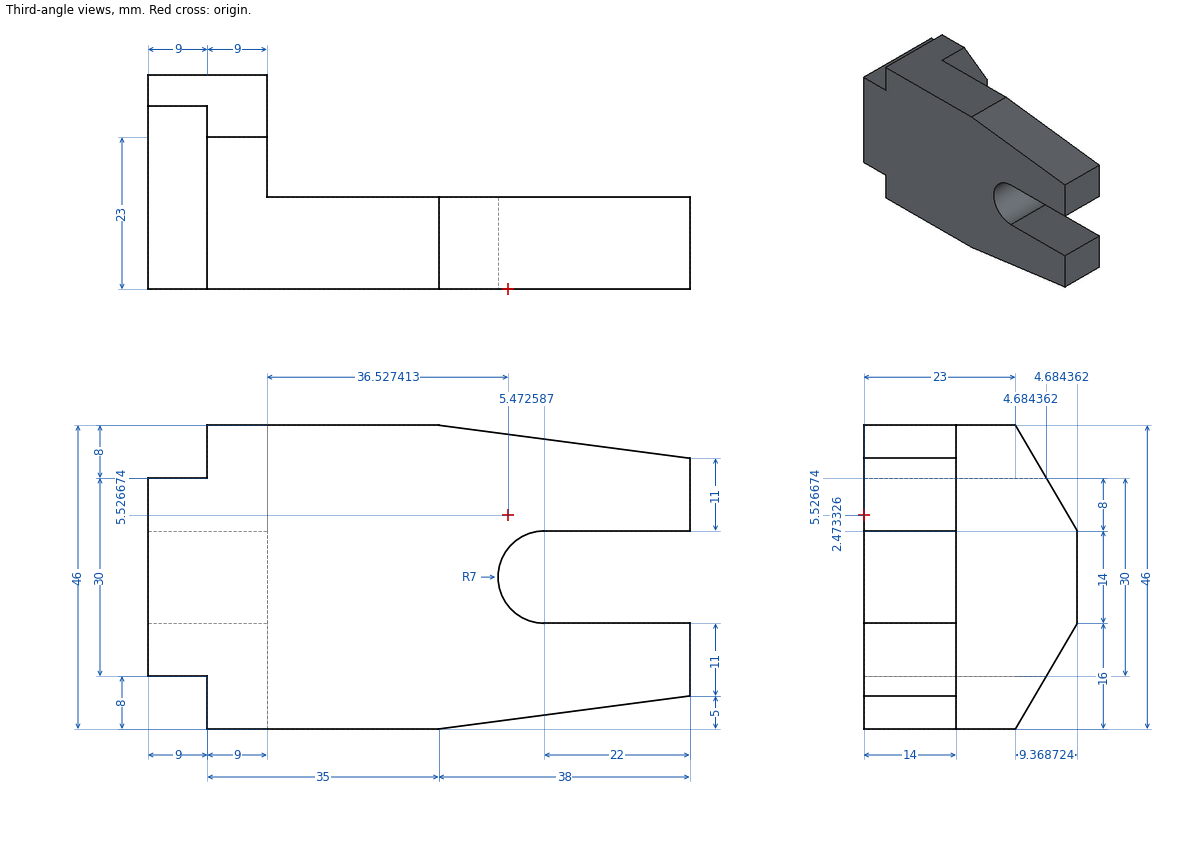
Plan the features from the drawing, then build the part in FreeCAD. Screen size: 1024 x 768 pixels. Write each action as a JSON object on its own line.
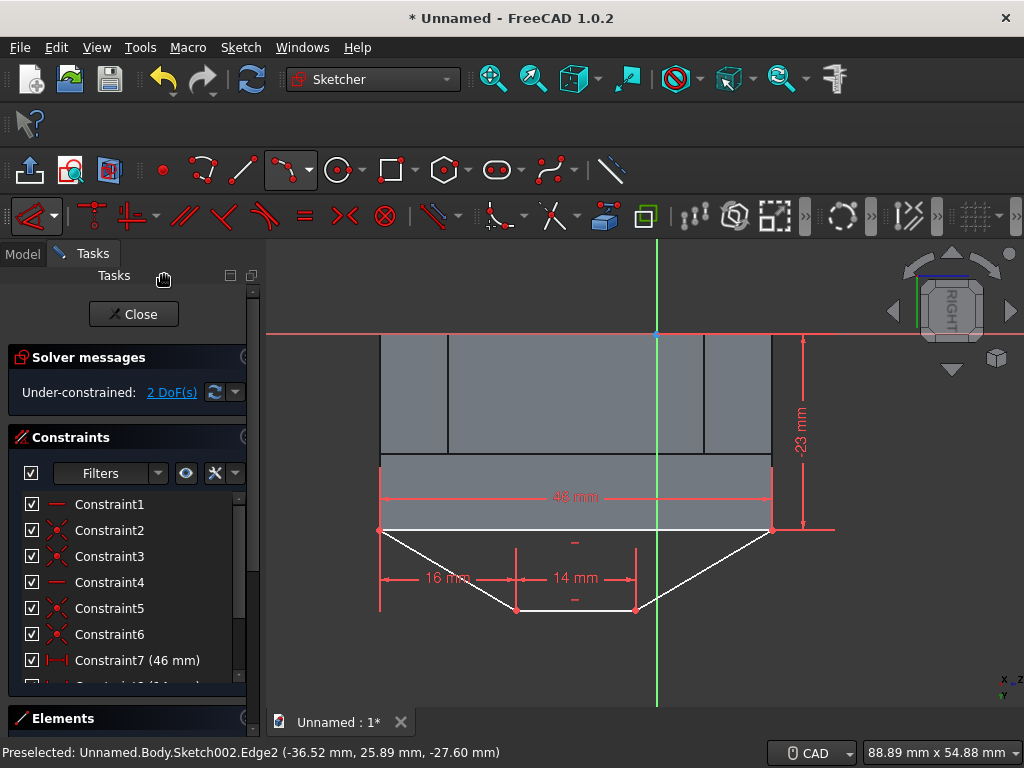
{"action": "scroll", "coordinate": [636, 611], "scroll_direction": "up", "scroll_amount": 4}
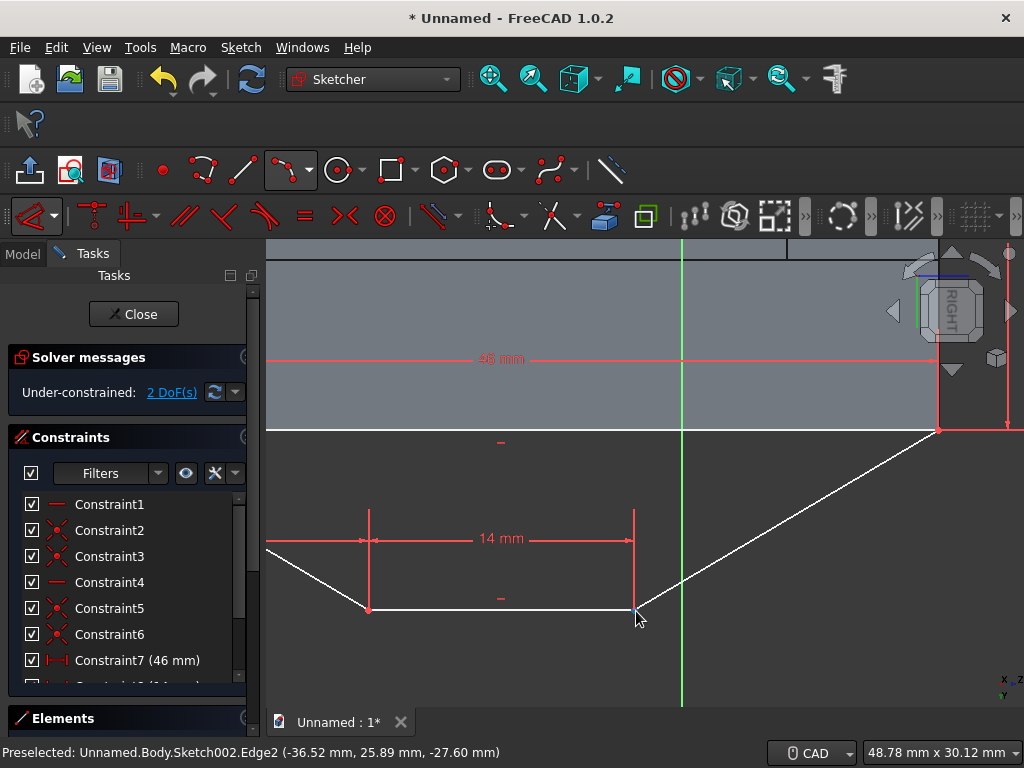
{"action": "left_click", "coordinate": [634, 610]}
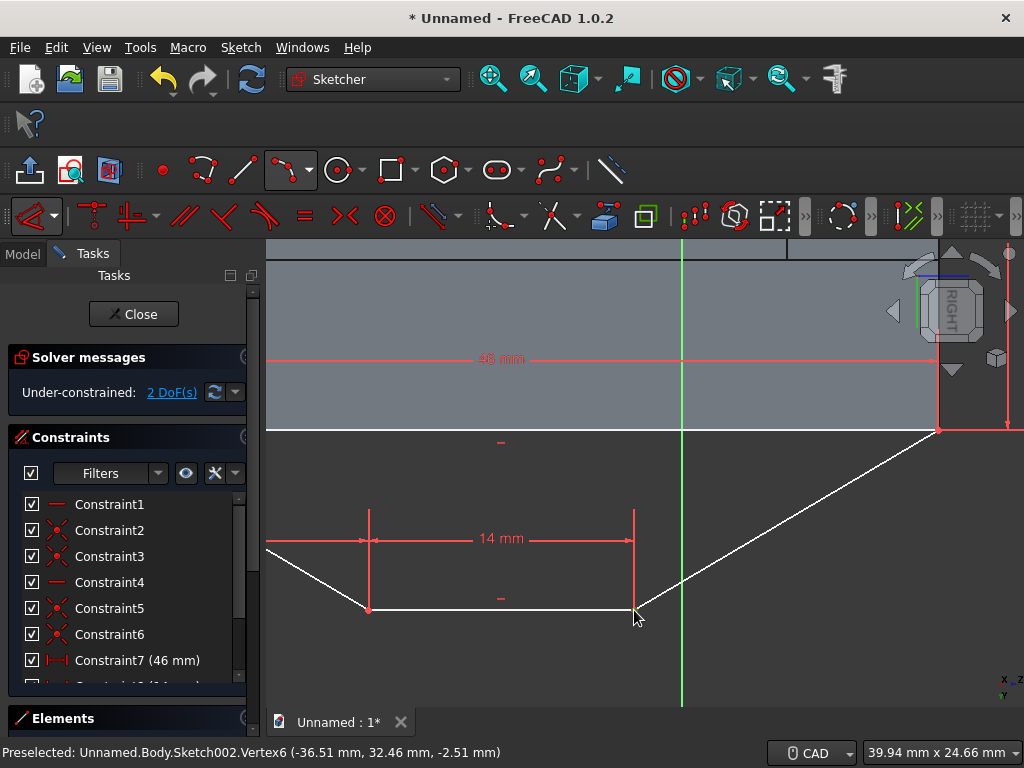
{"action": "left_click", "coordinate": [56, 216]}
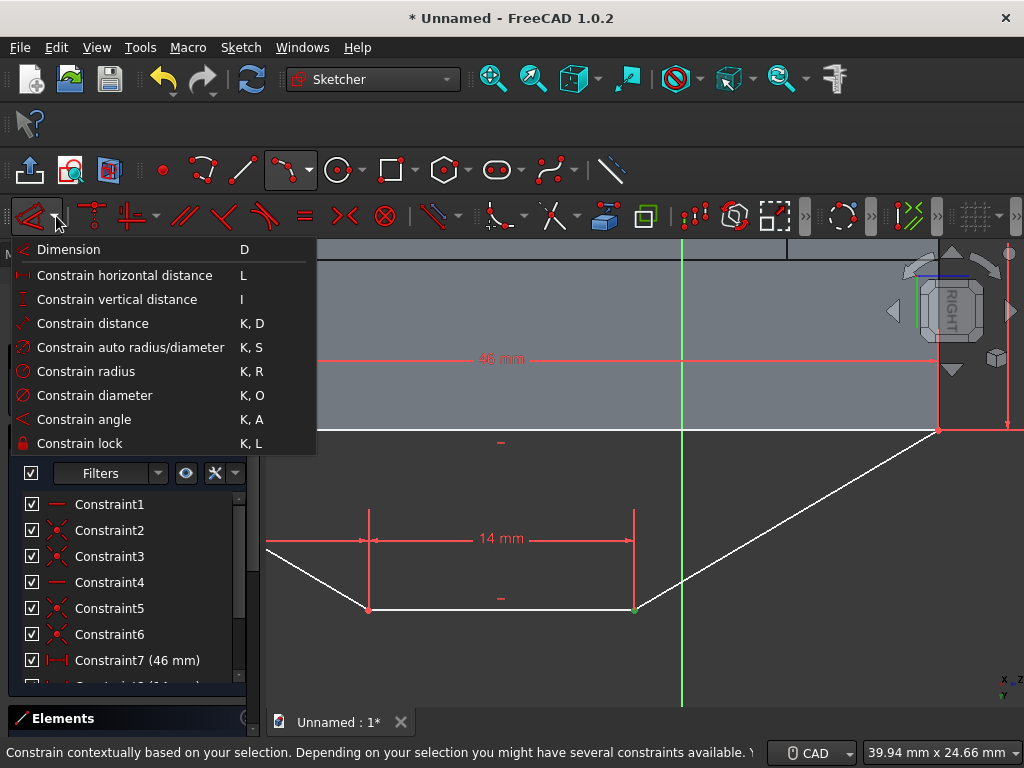
{"action": "left_click", "coordinate": [164, 275]}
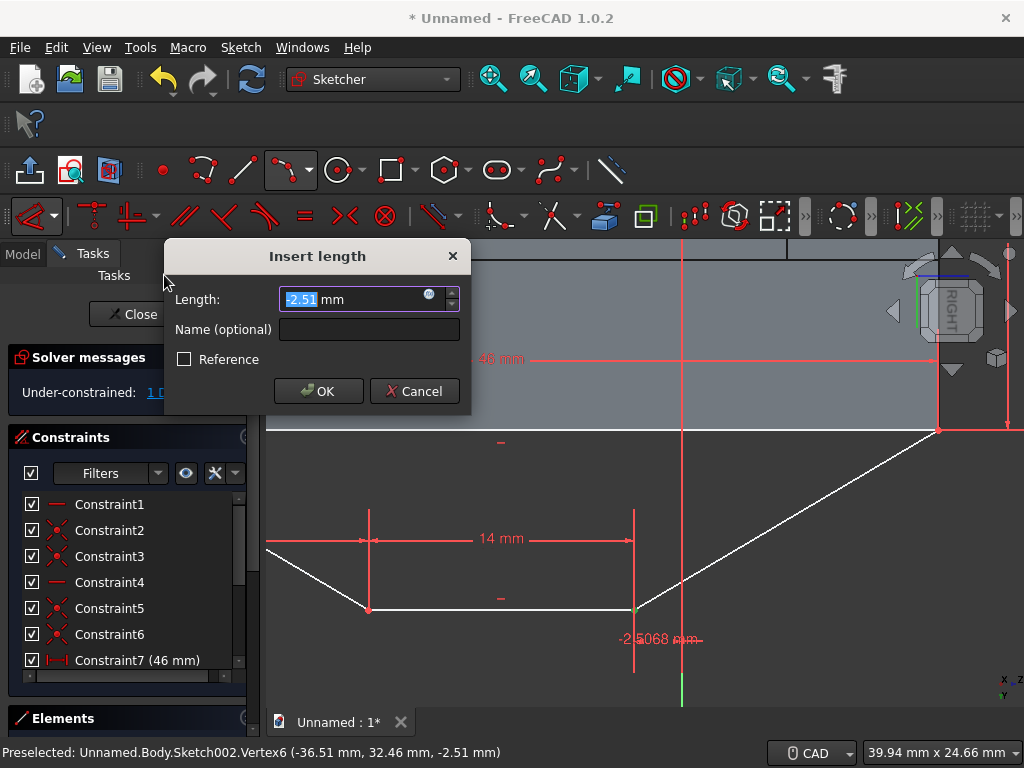
{"action": "type", "text": "-2.473326"}
{"action": "key", "text": "Return"}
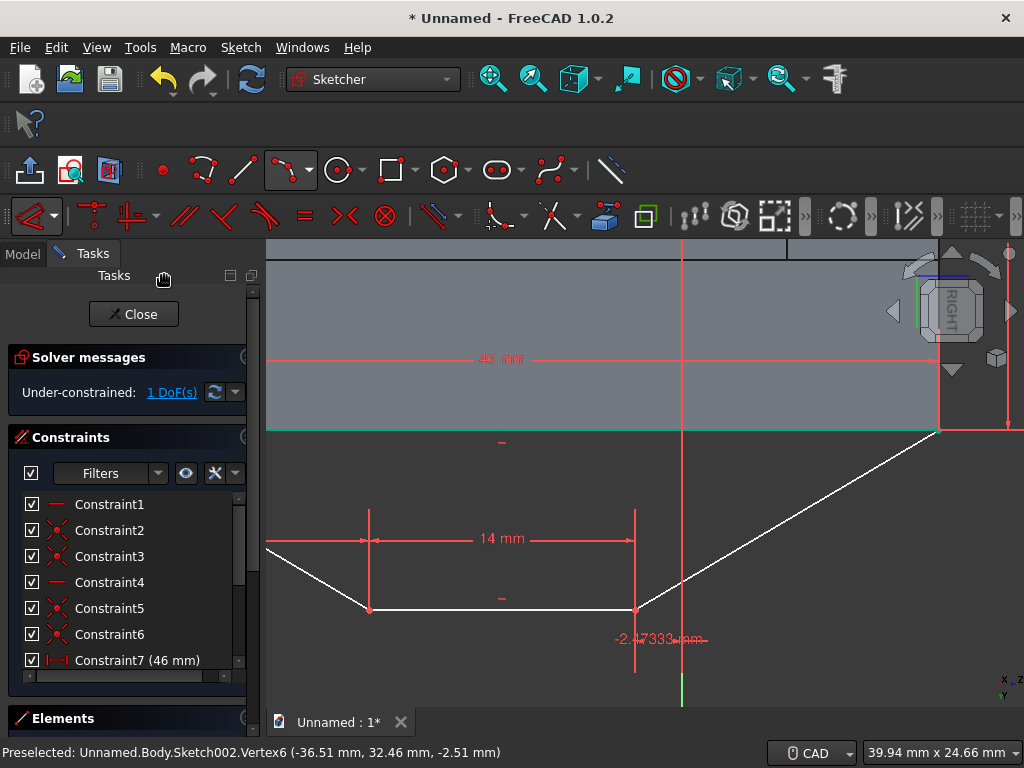
{"action": "left_click", "coordinate": [309, 574]}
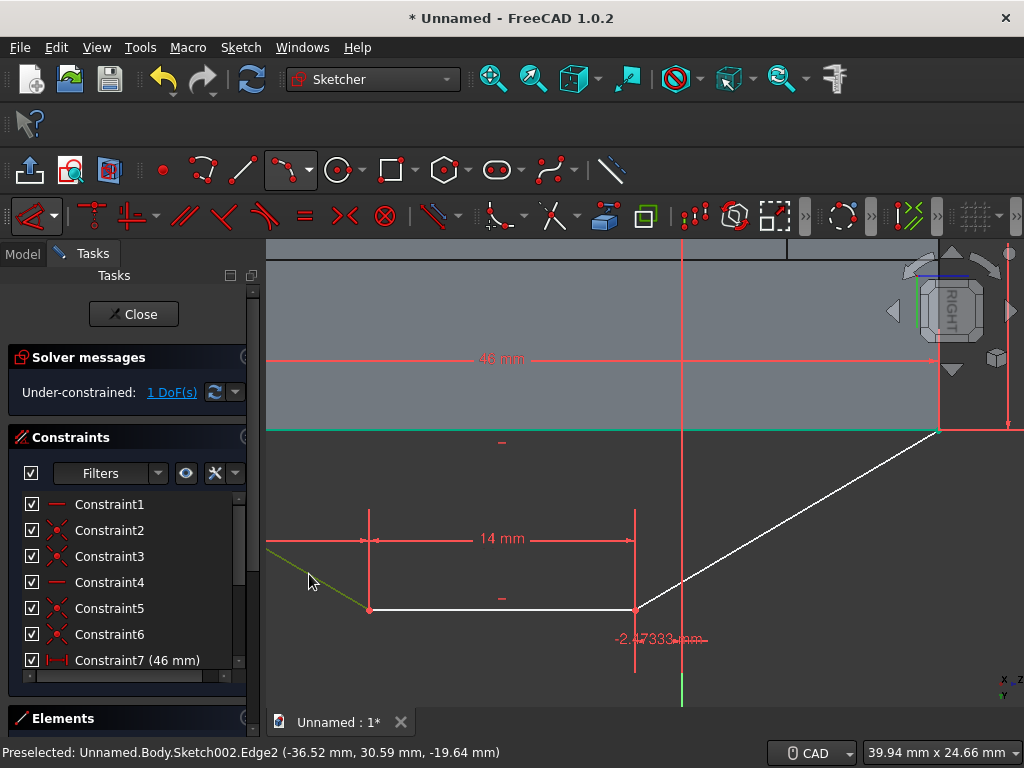
{"action": "key", "text": "i"}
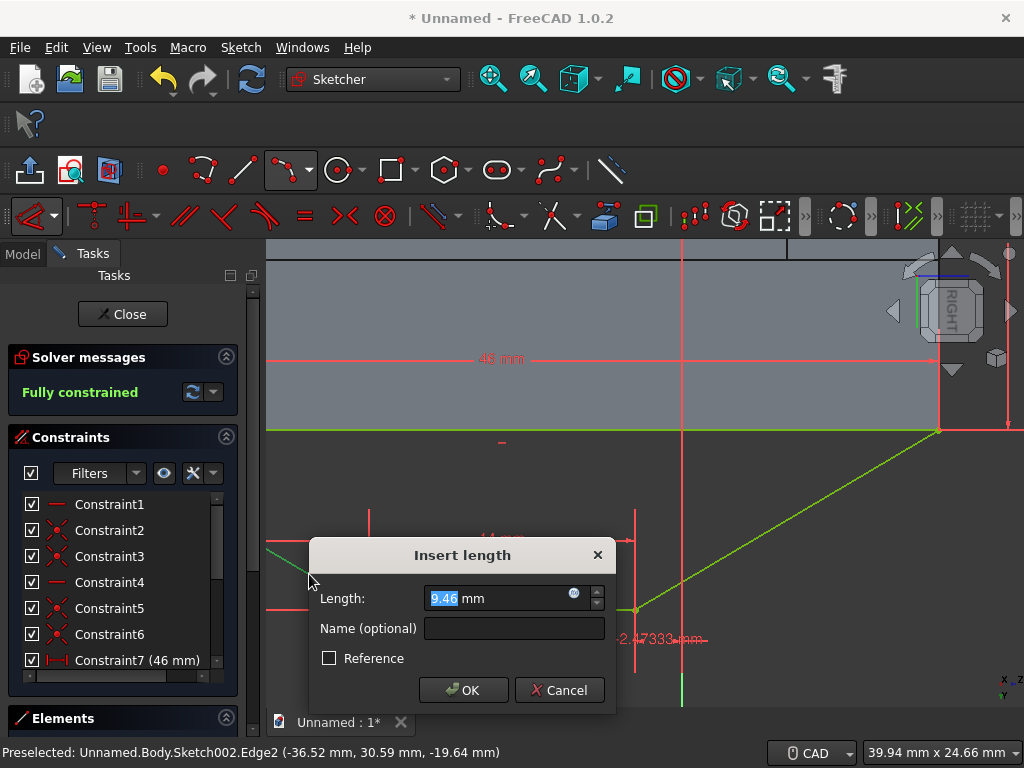
{"action": "type", "text": "9.368724"}
{"action": "key", "text": "Return"}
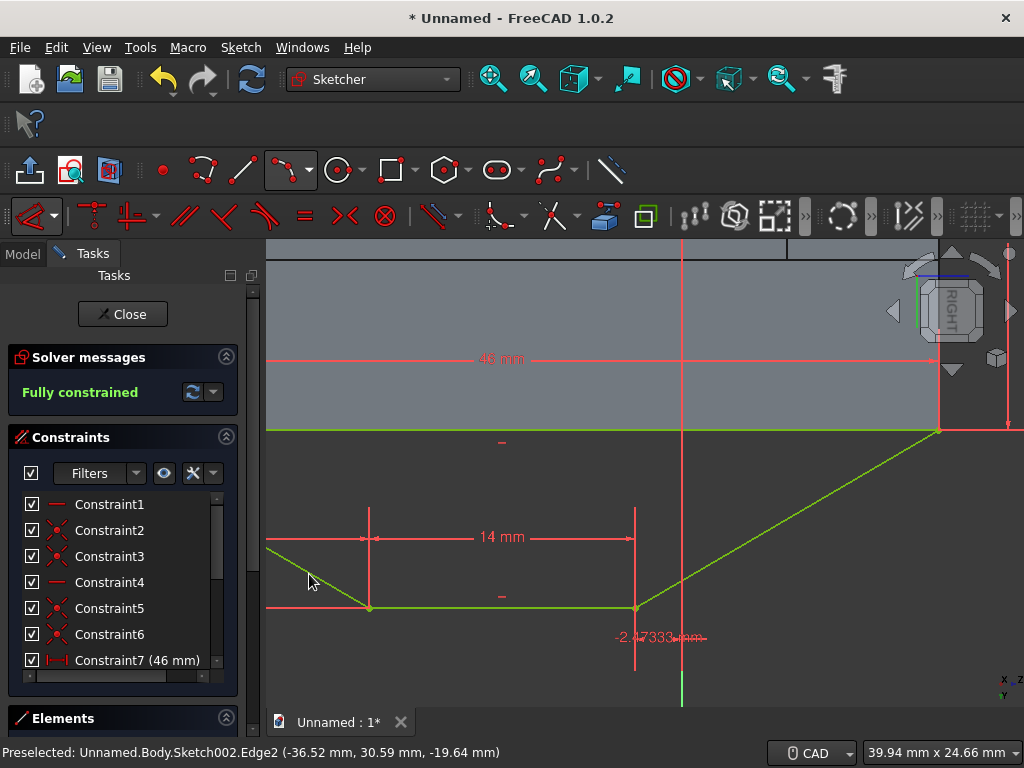
{"action": "left_click", "coordinate": [123, 314]}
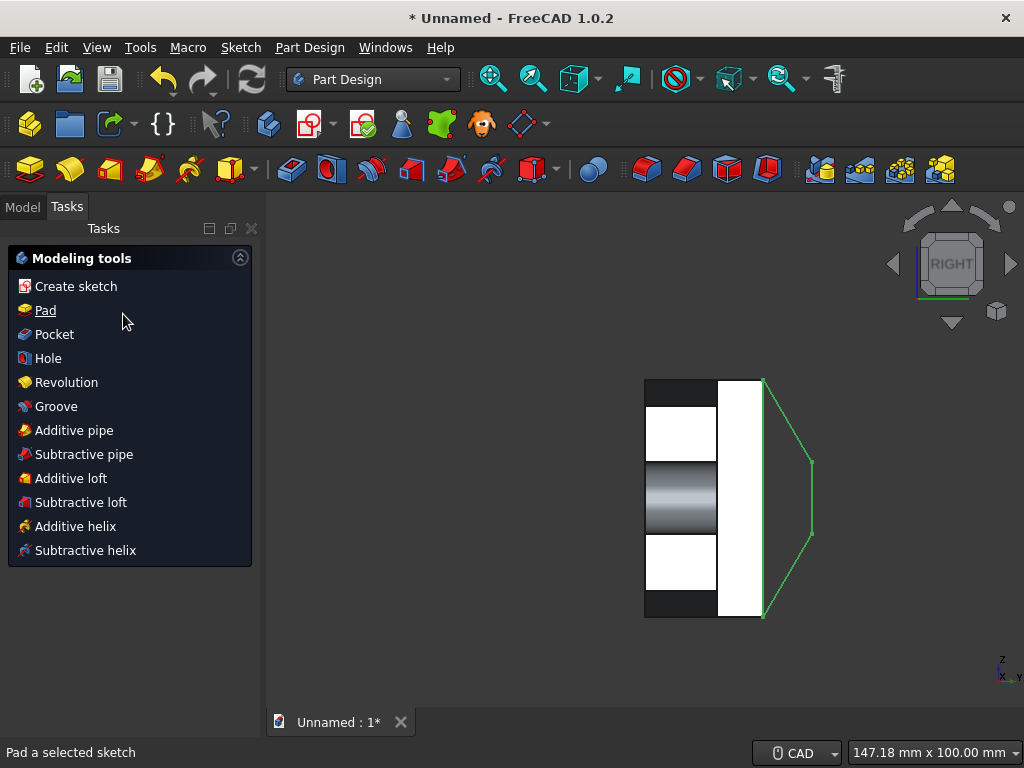
{"action": "left_click", "coordinate": [30, 170]}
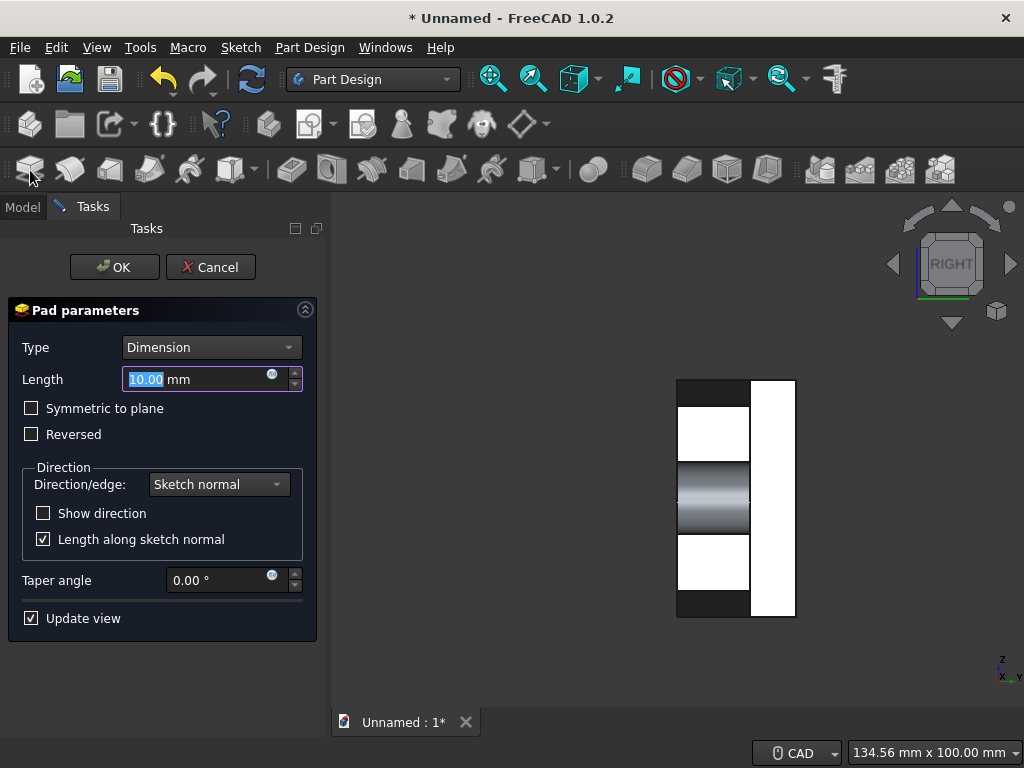
{"action": "type", "text": "9"}
{"action": "key", "text": "Tab"}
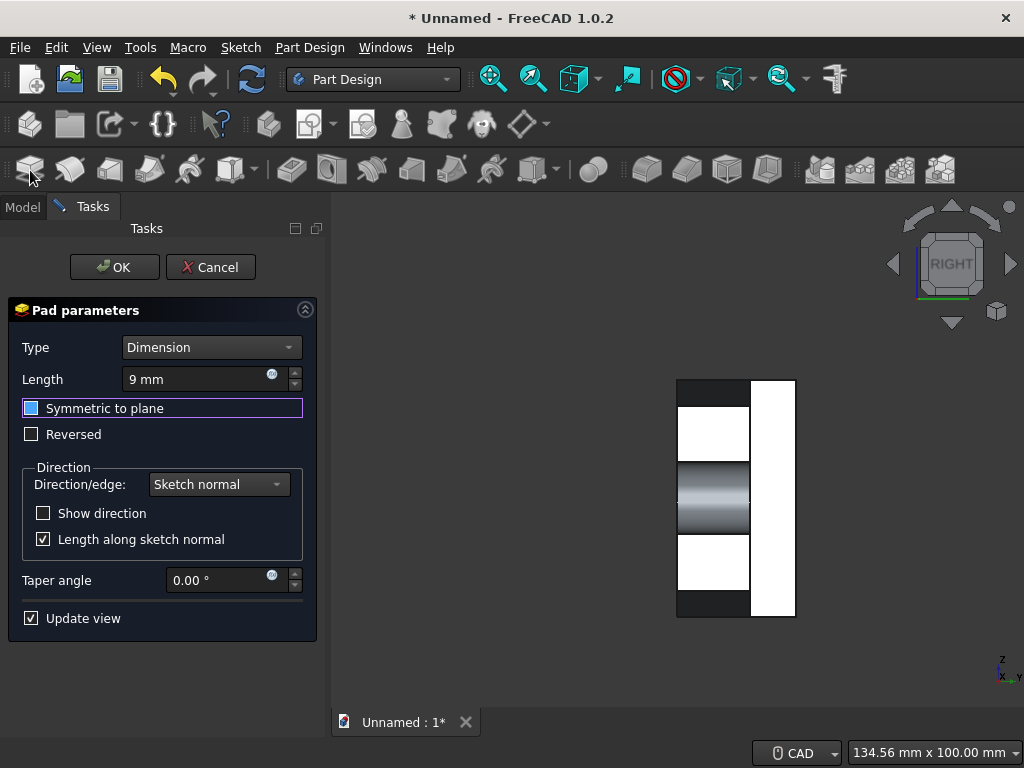
{"action": "left_click", "coordinate": [30, 434]}